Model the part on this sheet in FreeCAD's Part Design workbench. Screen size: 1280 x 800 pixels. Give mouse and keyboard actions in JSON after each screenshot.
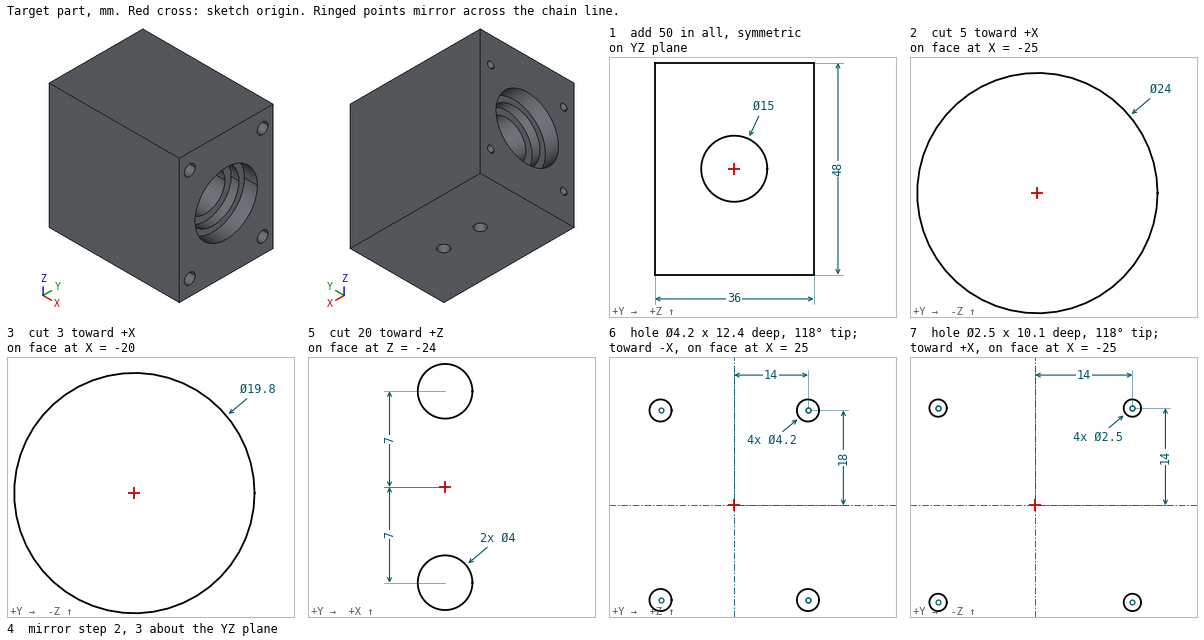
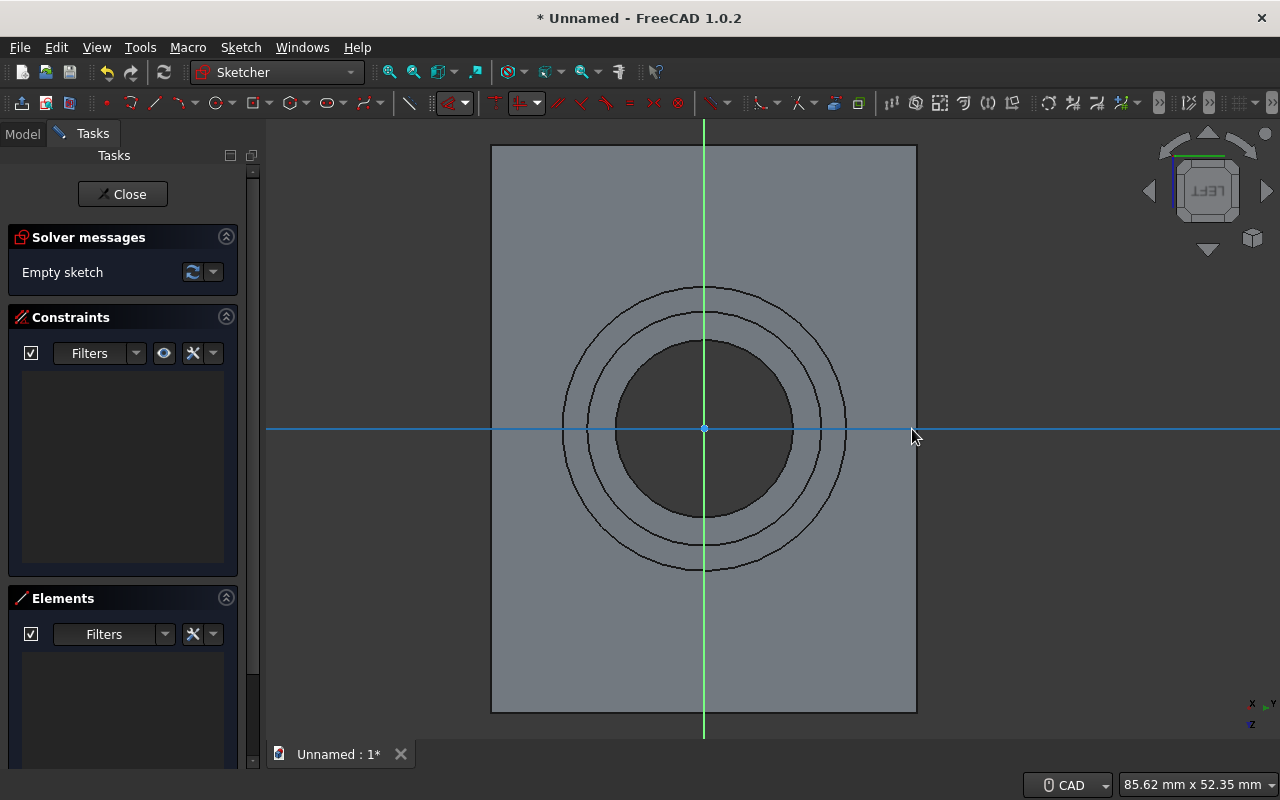
{"action": "left_click", "coordinate": [216, 104]}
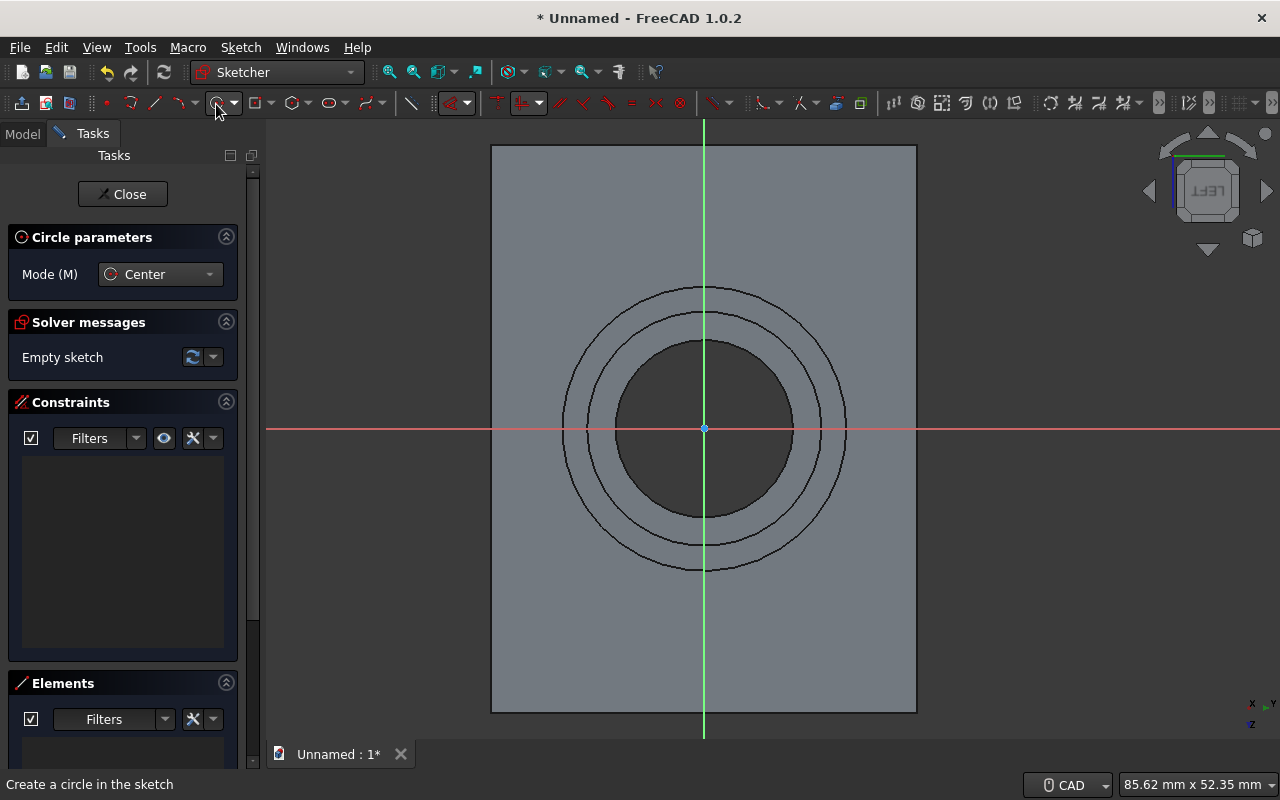
{"action": "scroll", "coordinate": [870, 263], "scroll_direction": "up", "scroll_amount": 3}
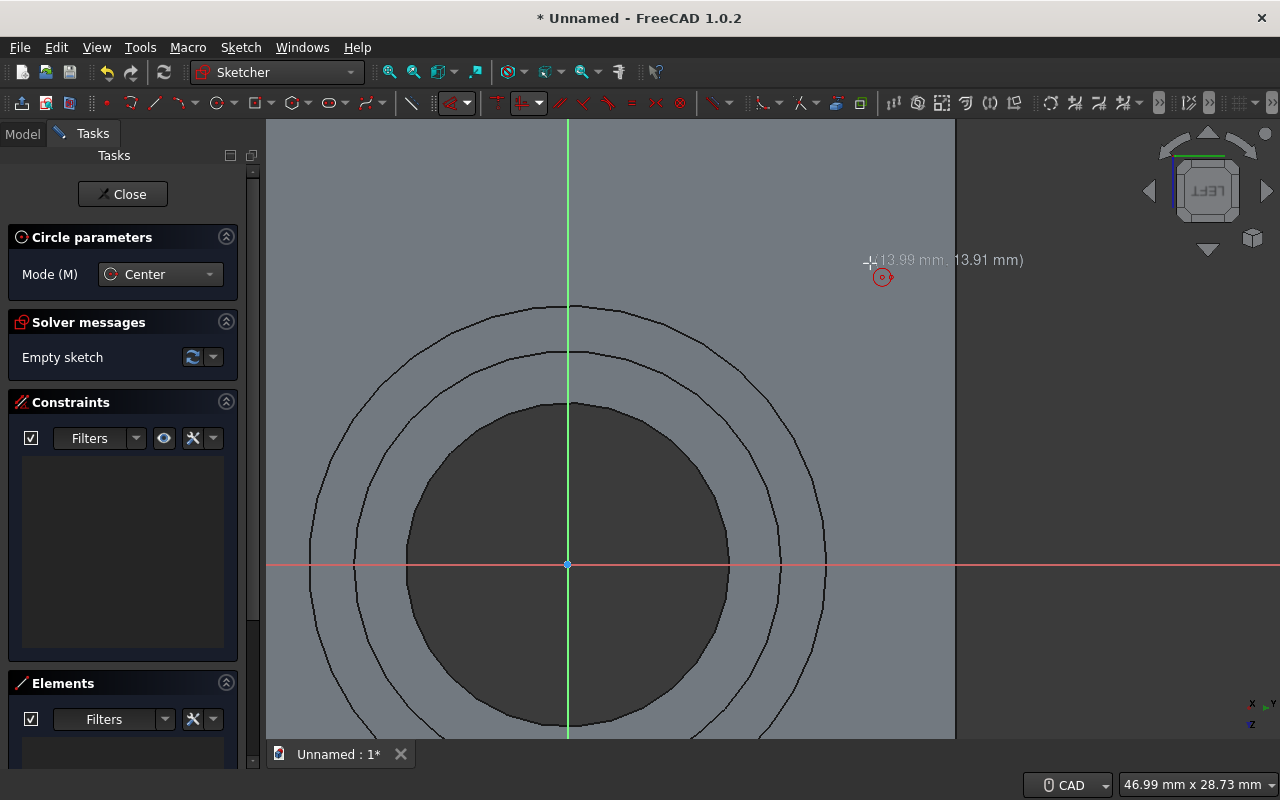
{"action": "left_click", "coordinate": [870, 263]}
{"action": "left_click", "coordinate": [889, 244]}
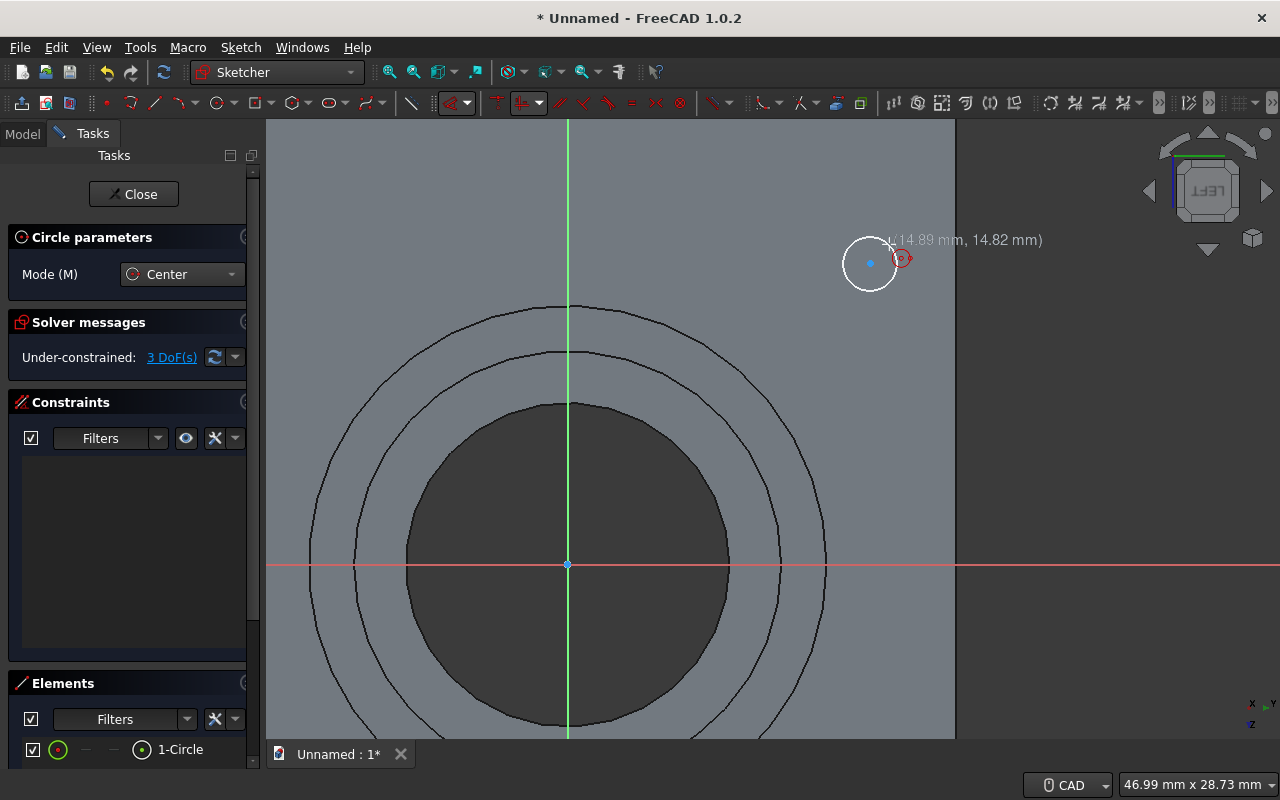
{"action": "scroll", "coordinate": [871, 264], "scroll_direction": "down", "scroll_amount": 3}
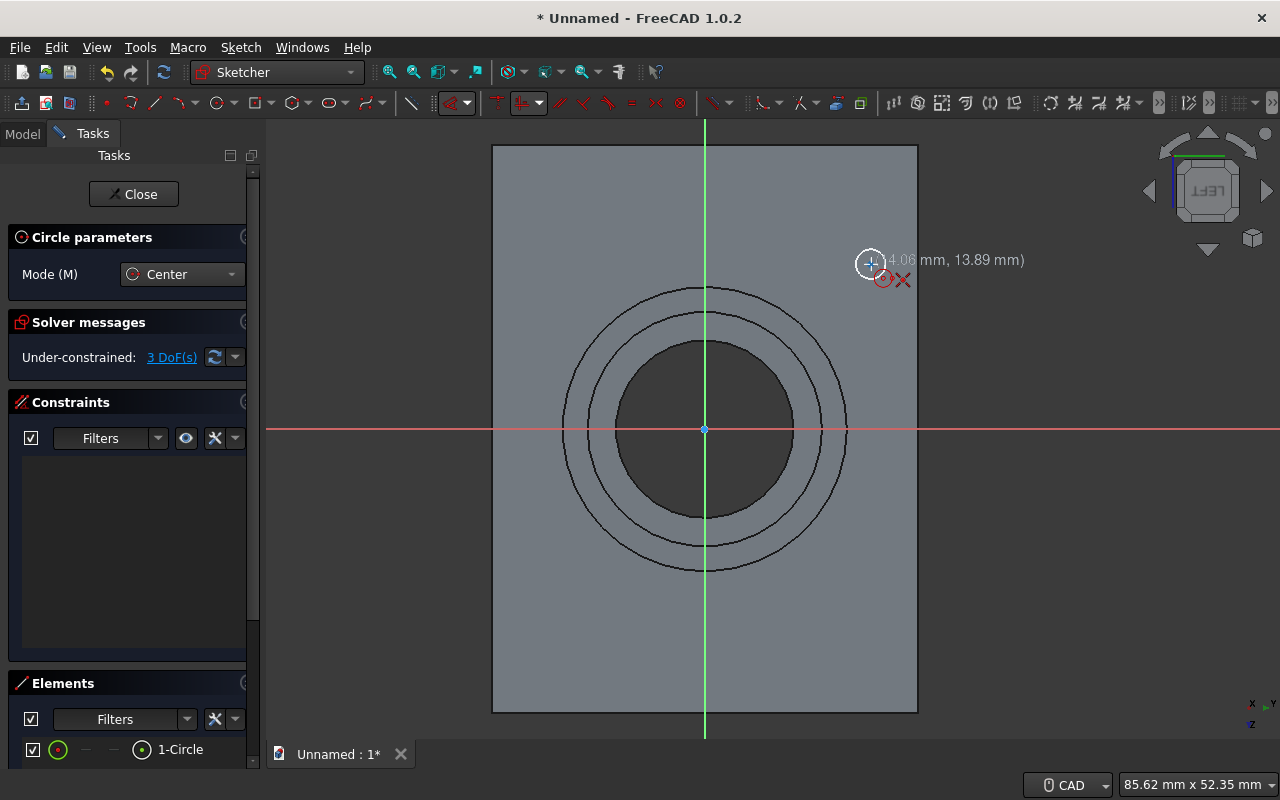
{"action": "scroll", "coordinate": [539, 263], "scroll_direction": "up", "scroll_amount": 3}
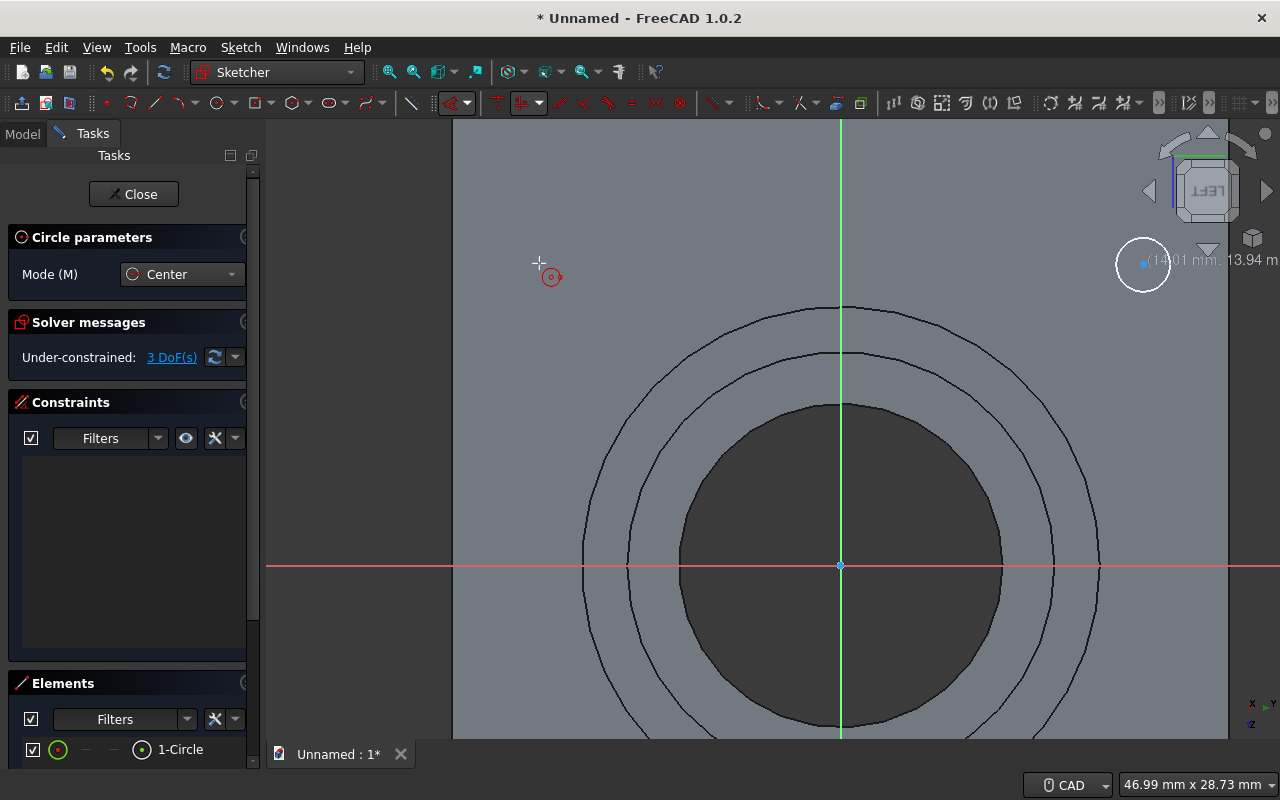
{"action": "left_click", "coordinate": [539, 264]}
{"action": "left_click", "coordinate": [558, 244]}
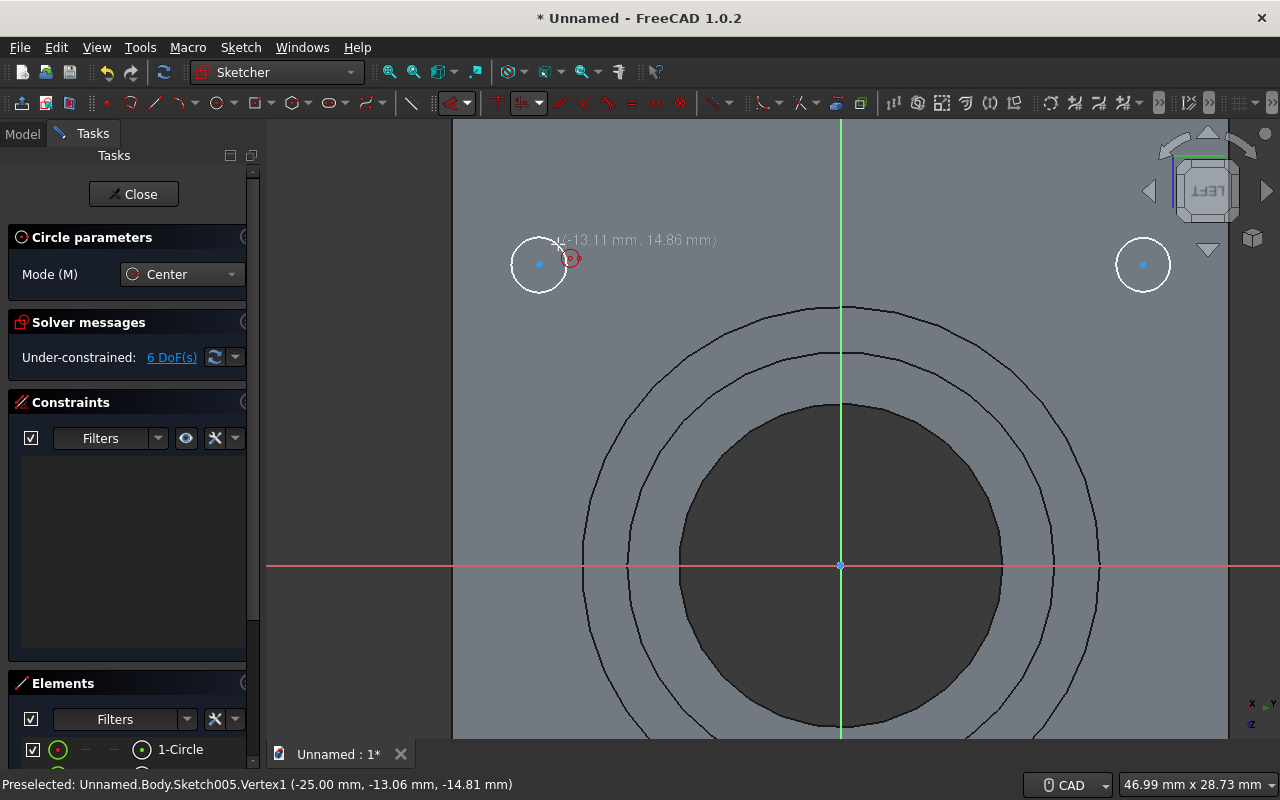
{"action": "scroll", "coordinate": [539, 263], "scroll_direction": "down", "scroll_amount": 3}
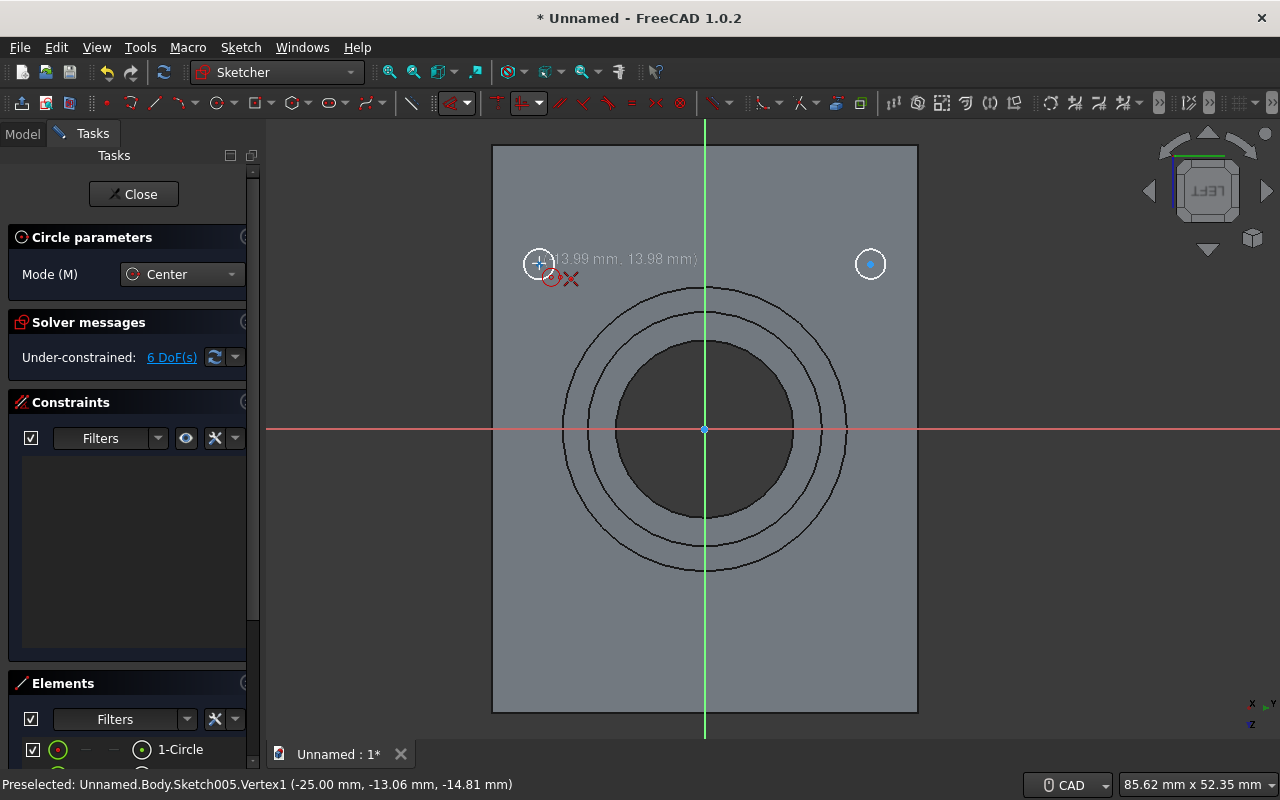
{"action": "scroll", "coordinate": [871, 595], "scroll_direction": "up", "scroll_amount": 3}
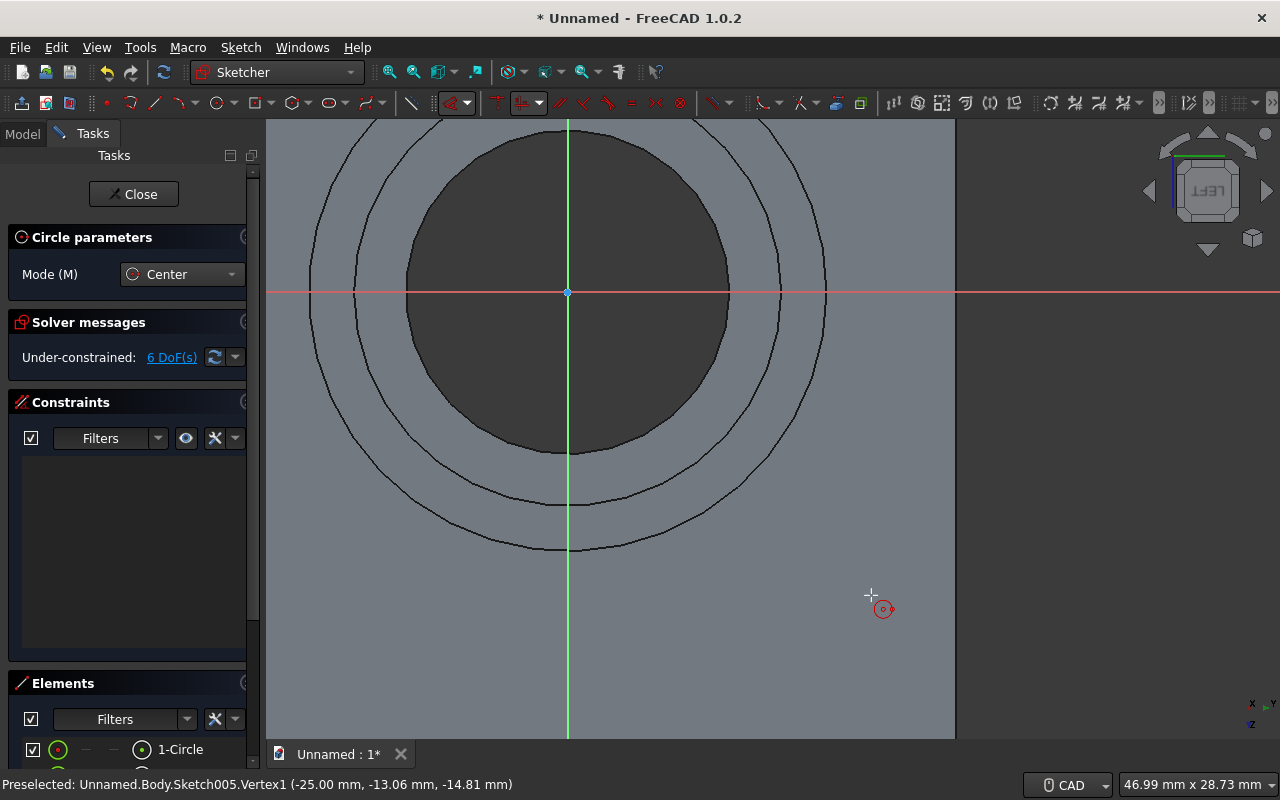
{"action": "left_click", "coordinate": [870, 594]}
{"action": "left_click", "coordinate": [889, 575]}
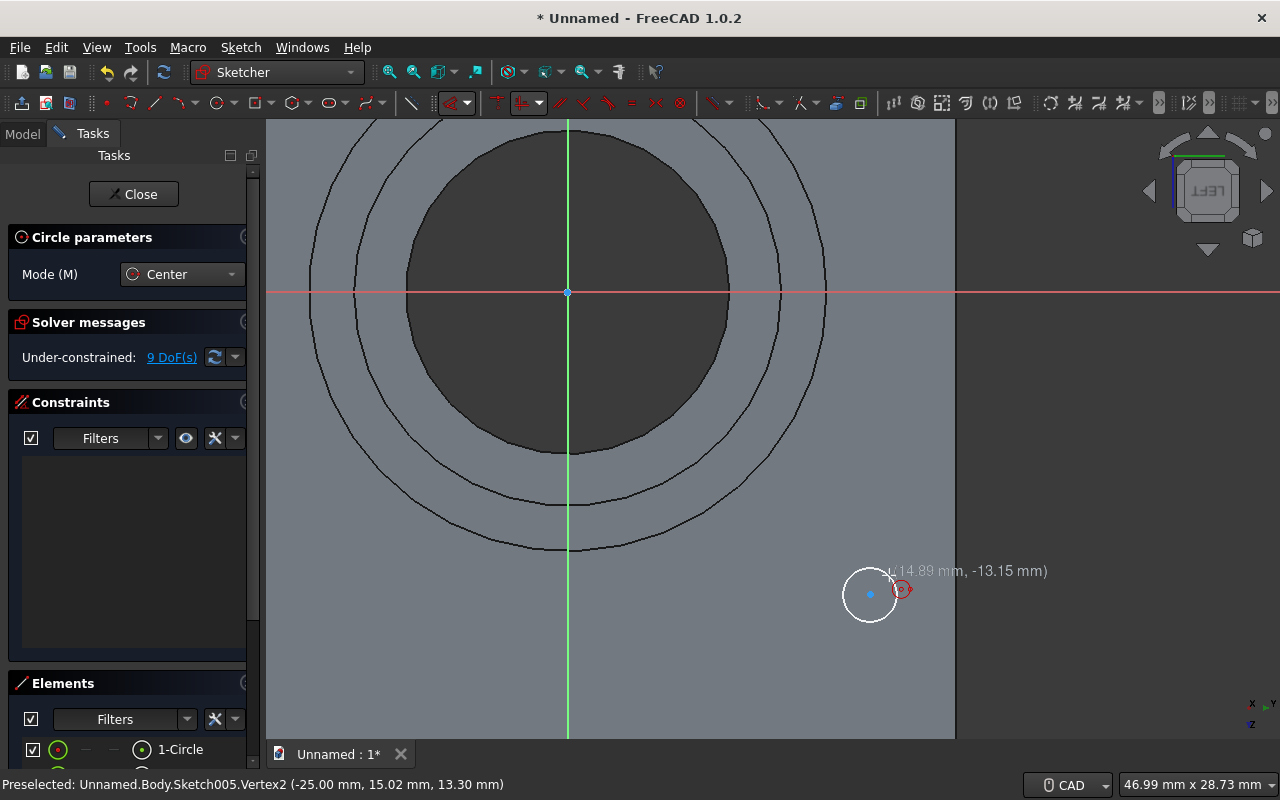
{"action": "scroll", "coordinate": [871, 595], "scroll_direction": "down", "scroll_amount": 3}